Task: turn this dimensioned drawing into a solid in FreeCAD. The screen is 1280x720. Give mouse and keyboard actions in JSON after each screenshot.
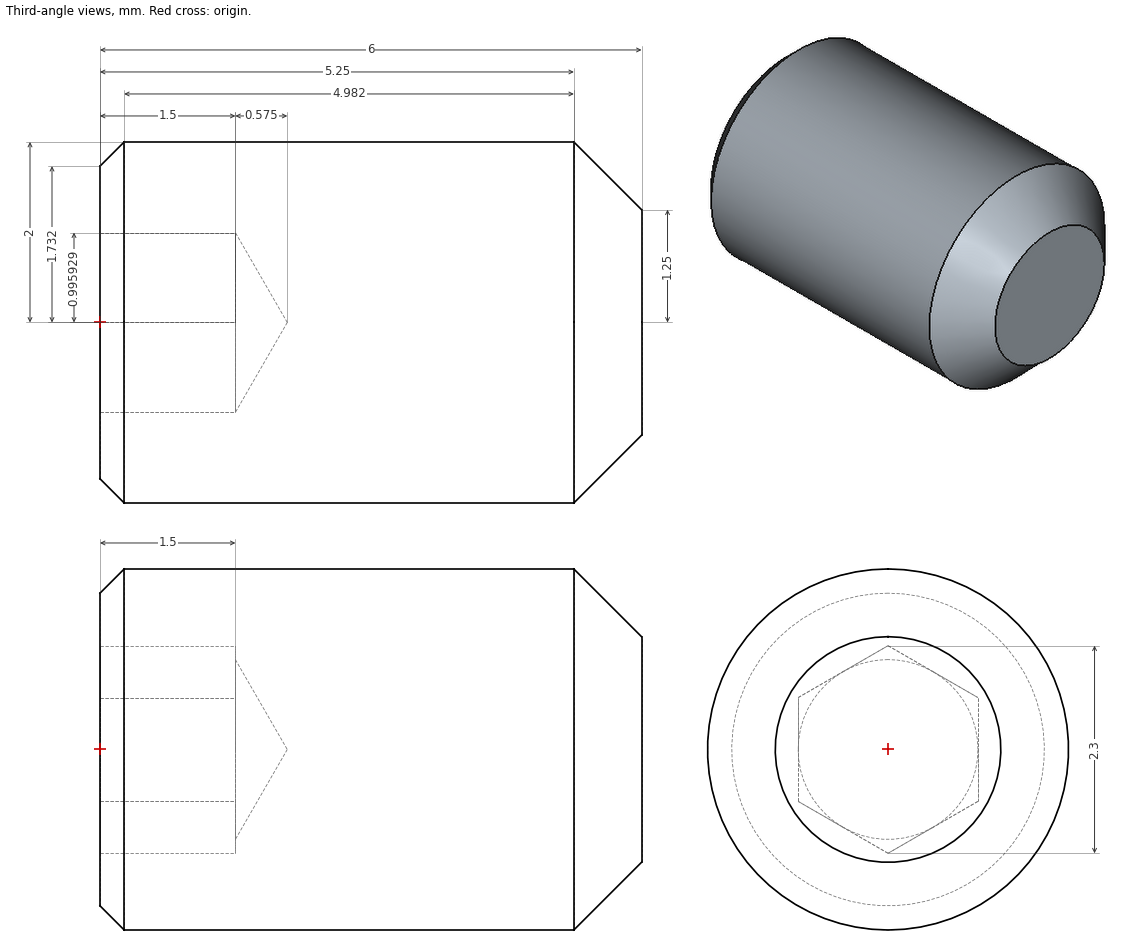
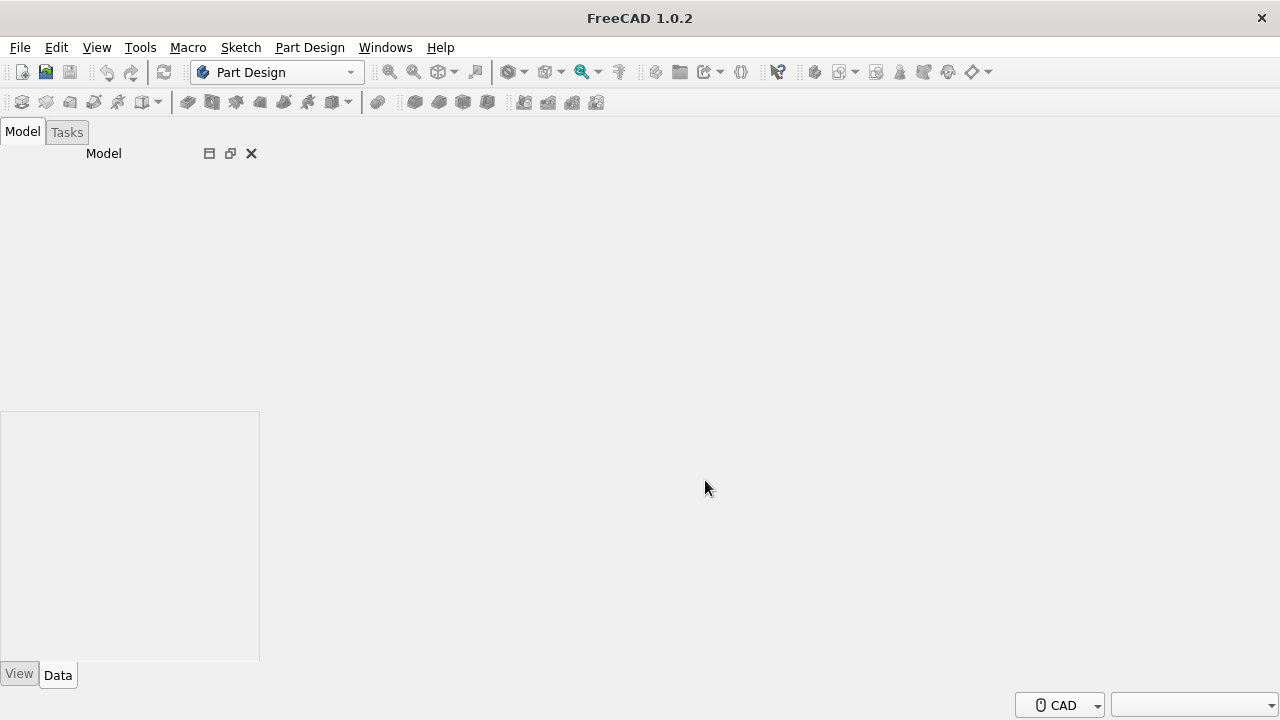
{"action": "left_click", "coordinate": [22, 72]}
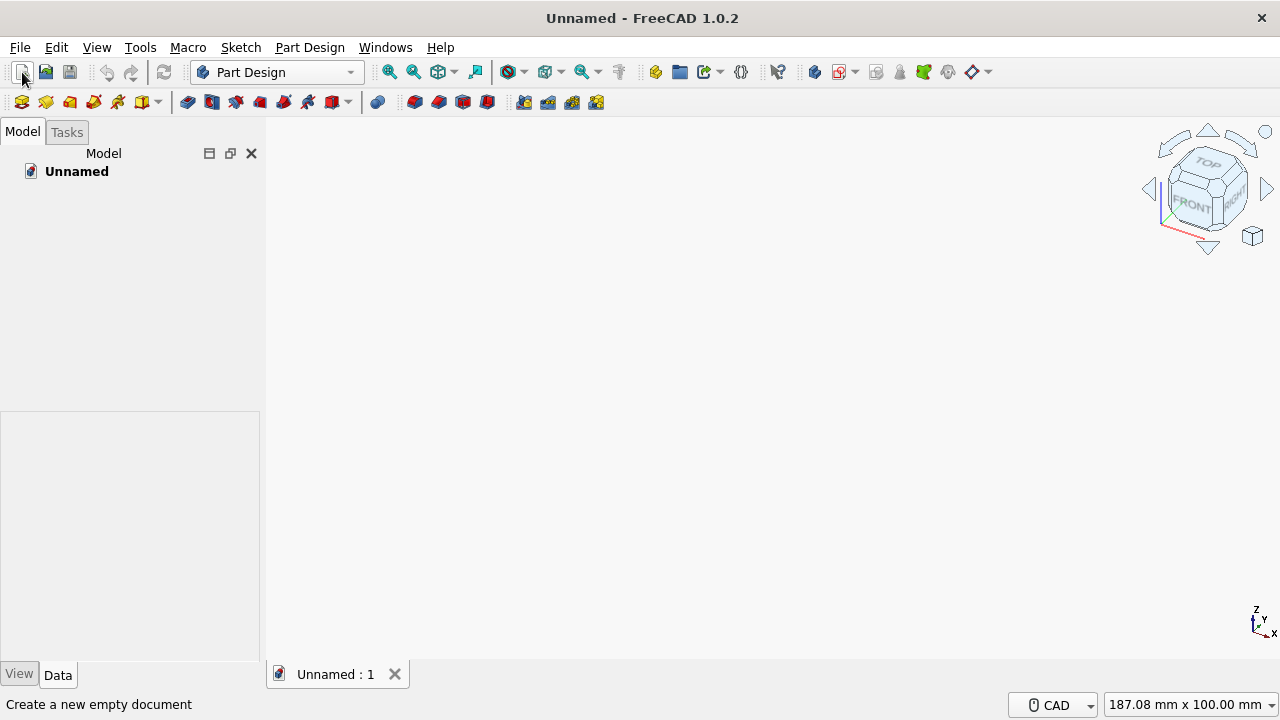
{"action": "left_click", "coordinate": [840, 72]}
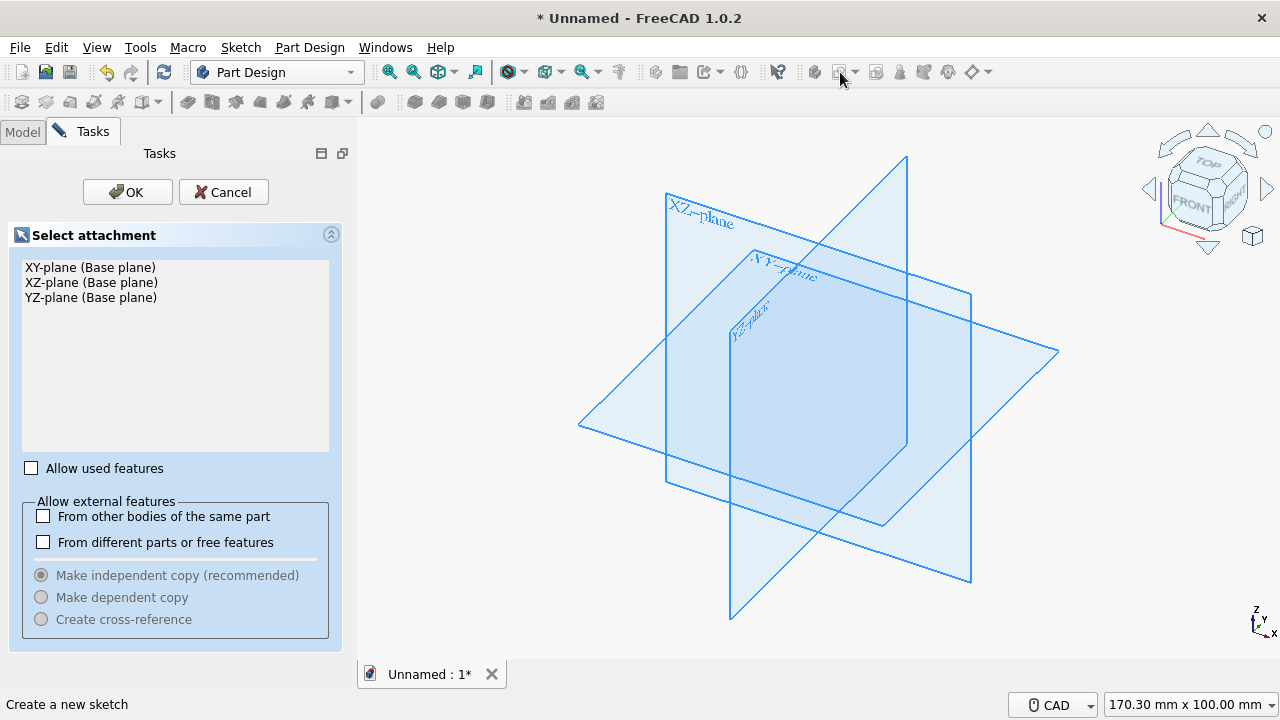
{"action": "left_click", "coordinate": [82, 268]}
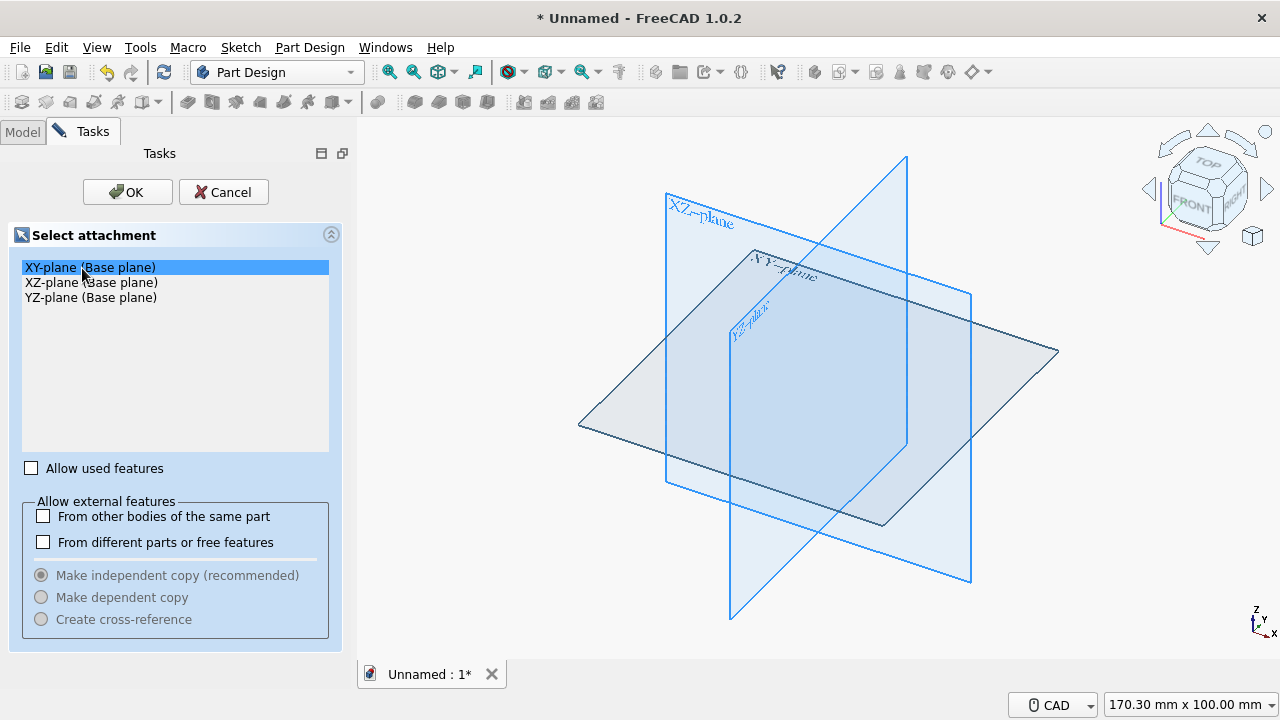
{"action": "left_click", "coordinate": [128, 192]}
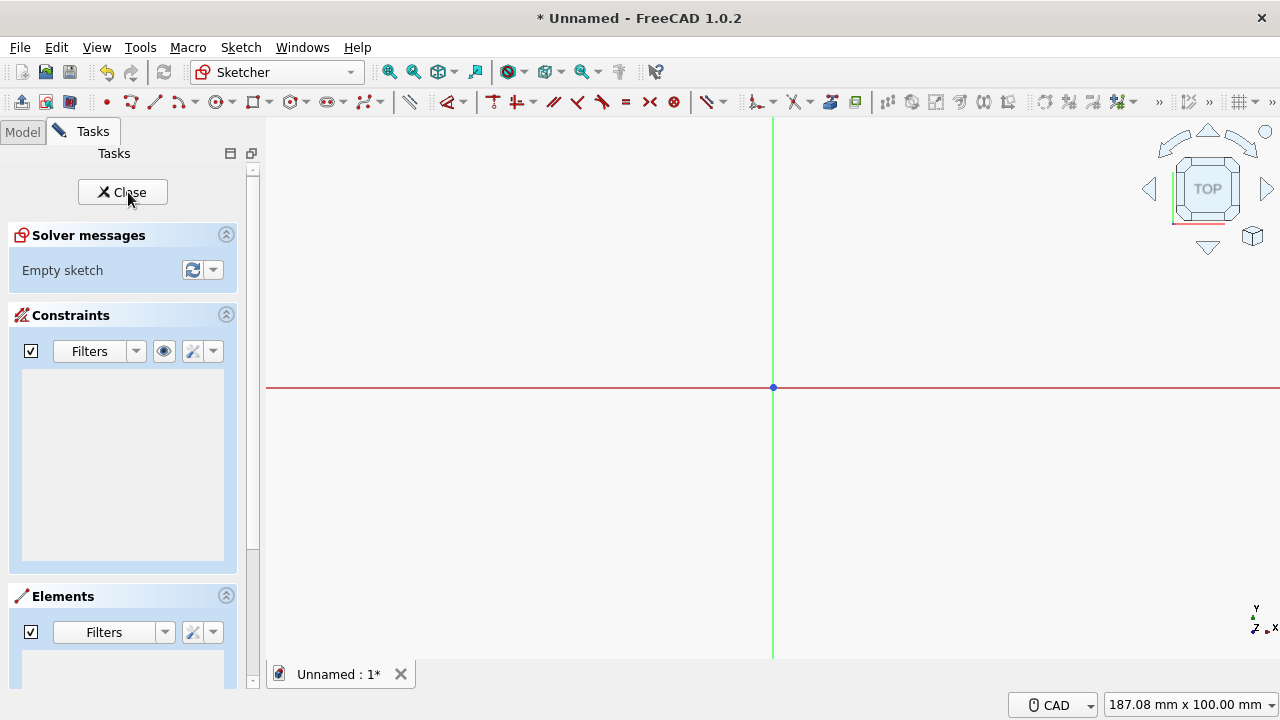
{"action": "scroll", "coordinate": [795, 382], "scroll_direction": "up", "scroll_amount": 14}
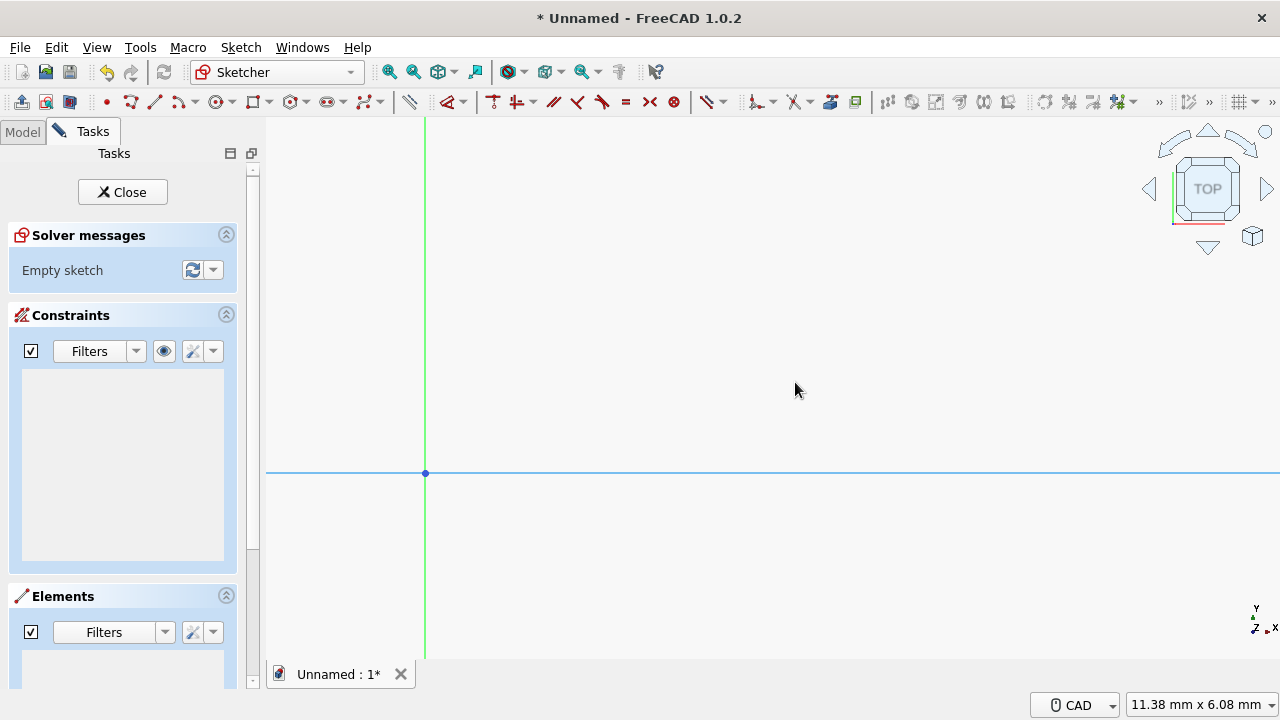
{"action": "left_click", "coordinate": [132, 102]}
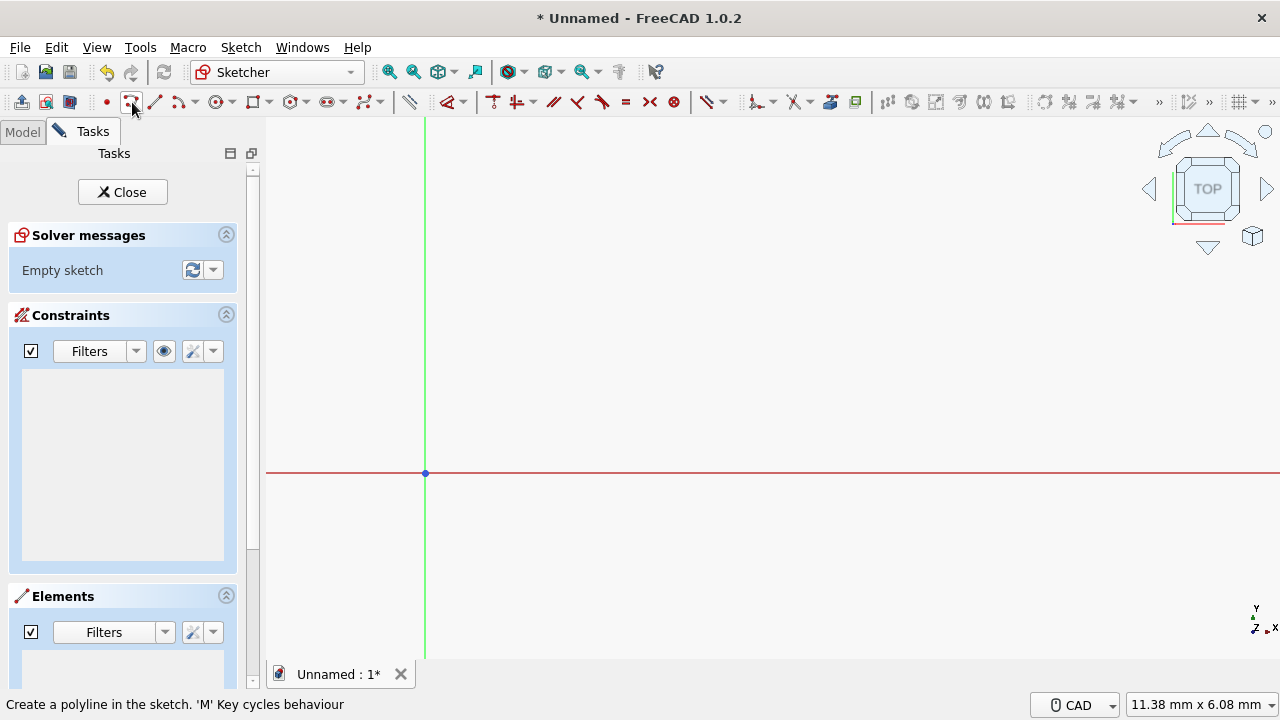
{"action": "left_click", "coordinate": [425, 473]}
{"action": "left_click", "coordinate": [960, 464]}
{"action": "left_click", "coordinate": [960, 362]}
{"action": "left_click", "coordinate": [893, 295]}
{"action": "left_click", "coordinate": [449, 295]}
{"action": "left_click", "coordinate": [434, 319]}
{"action": "left_click", "coordinate": [425, 473]}
{"action": "key", "text": "Escape"}
{"action": "key", "text": "Escape"}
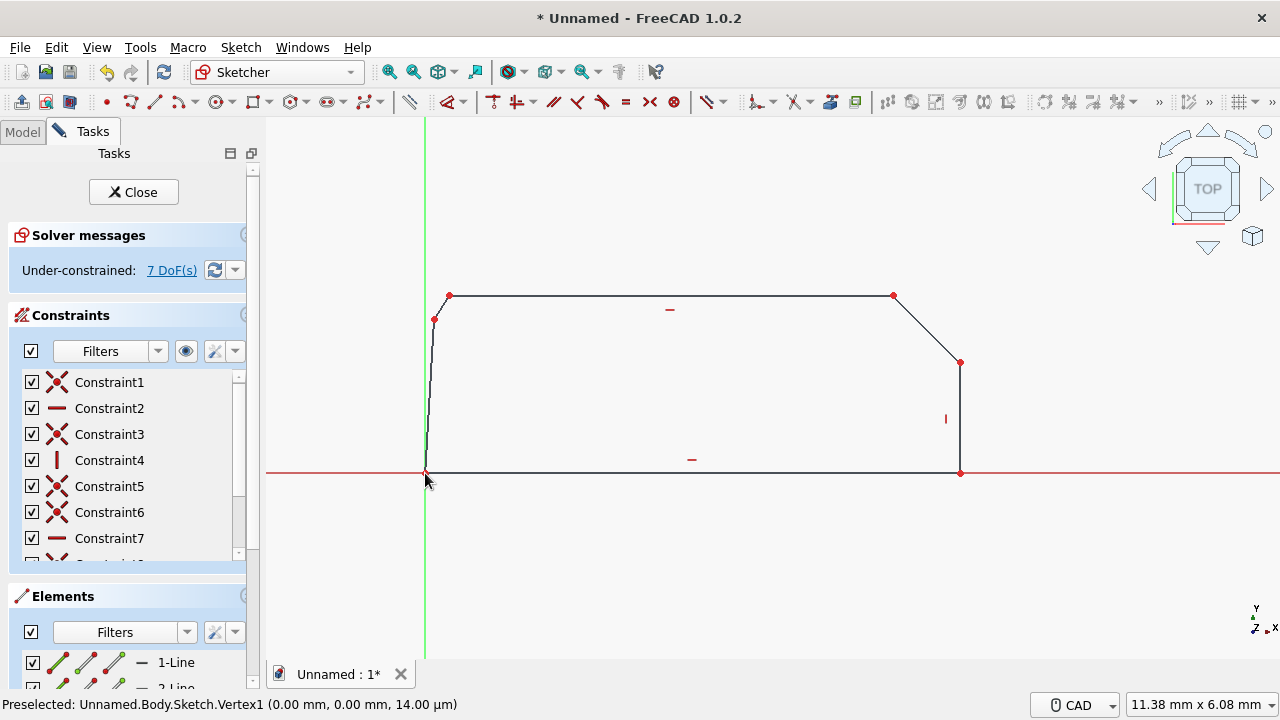
{"action": "left_click", "coordinate": [428, 427]}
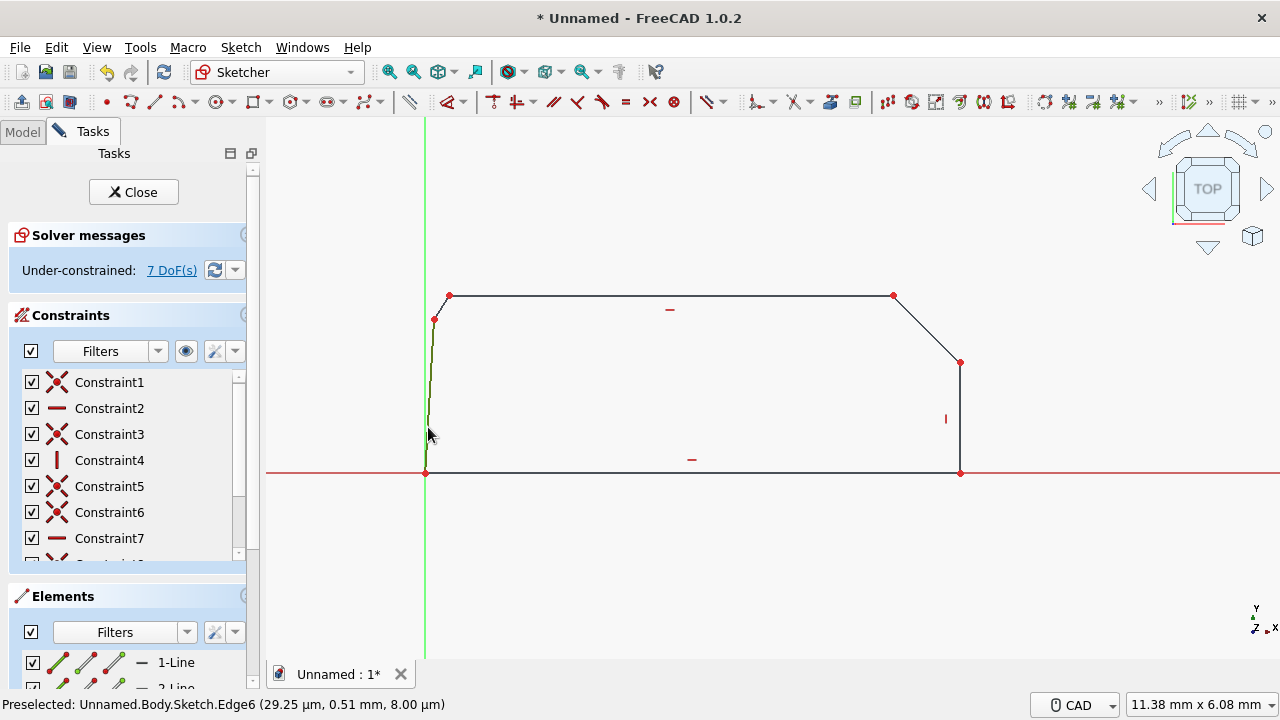
{"action": "left_click", "coordinate": [536, 102]}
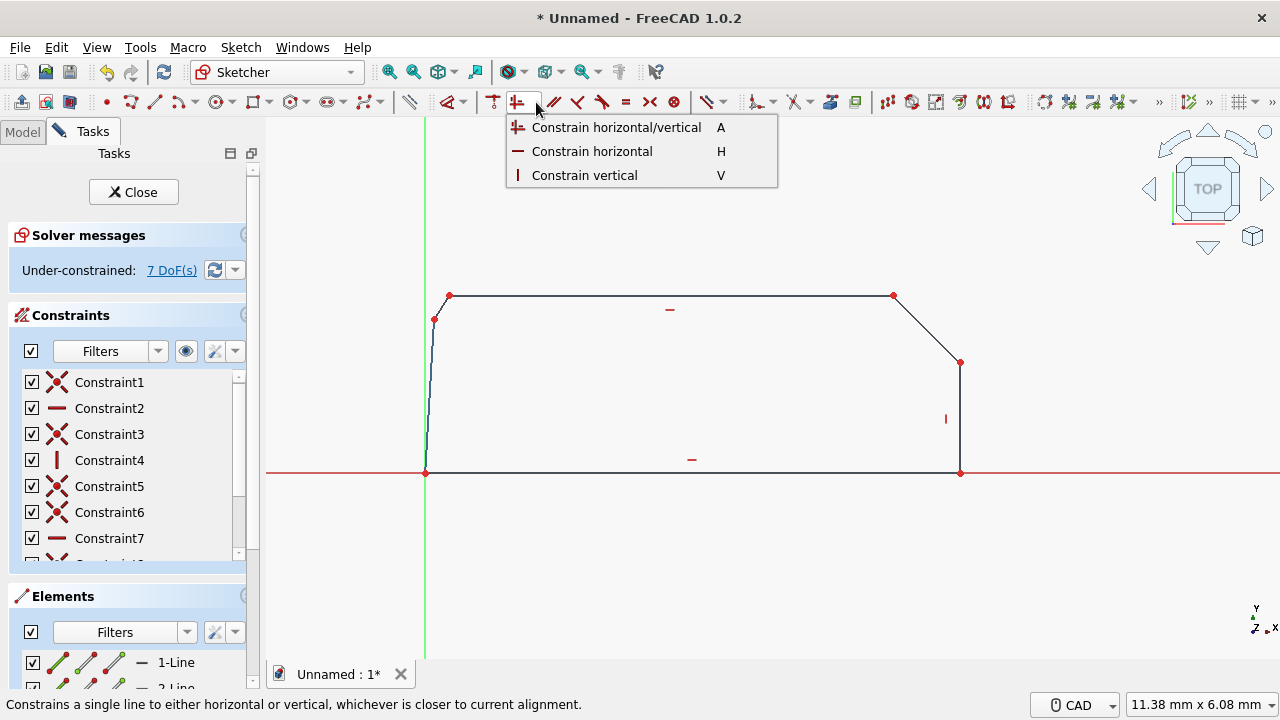
{"action": "left_click", "coordinate": [642, 175]}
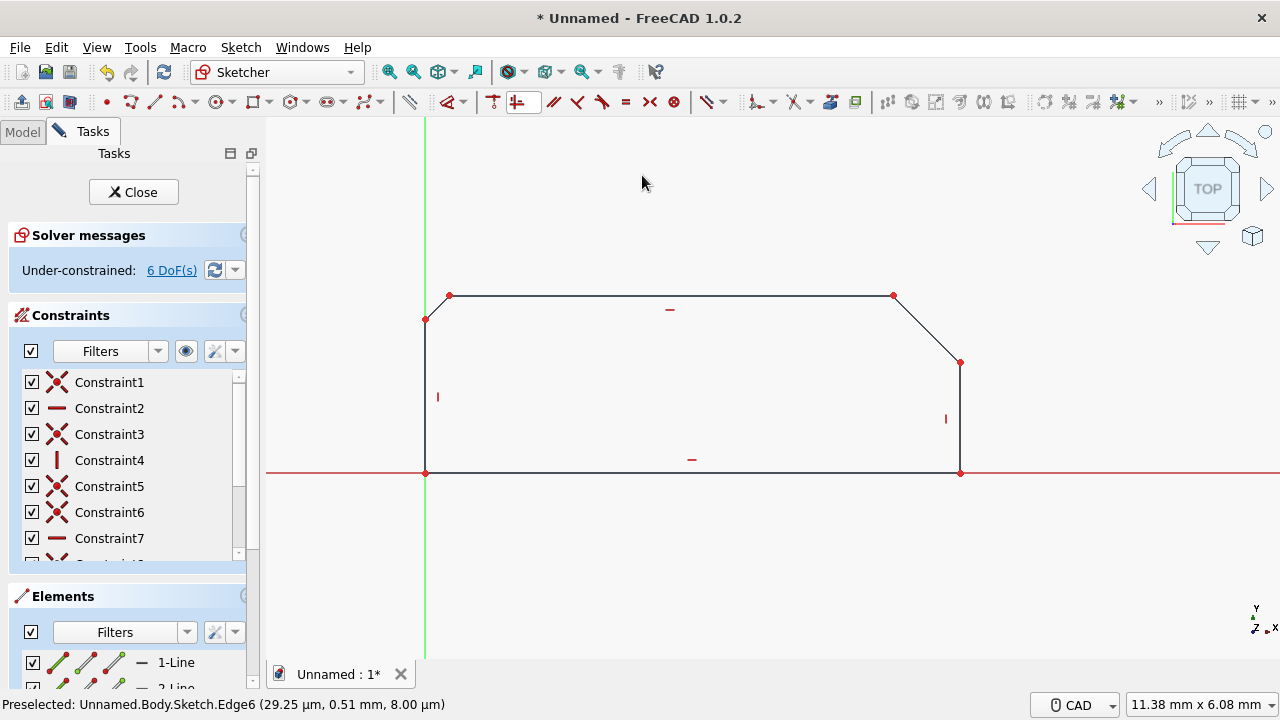
{"action": "left_click", "coordinate": [448, 102]}